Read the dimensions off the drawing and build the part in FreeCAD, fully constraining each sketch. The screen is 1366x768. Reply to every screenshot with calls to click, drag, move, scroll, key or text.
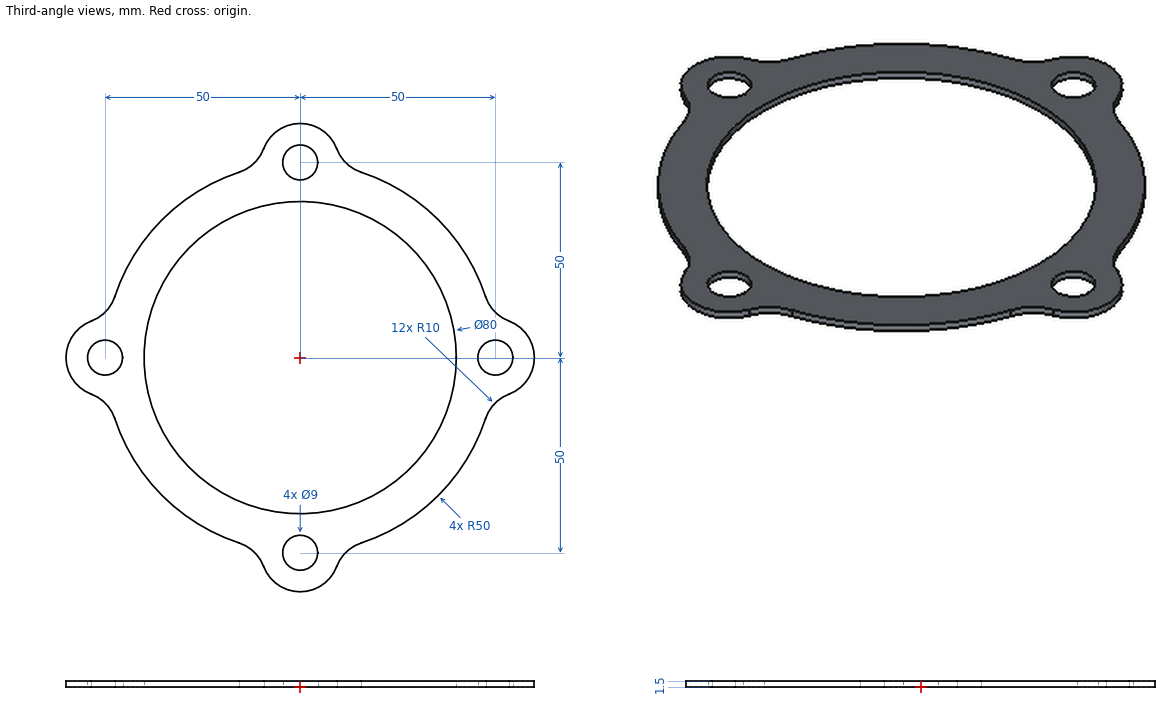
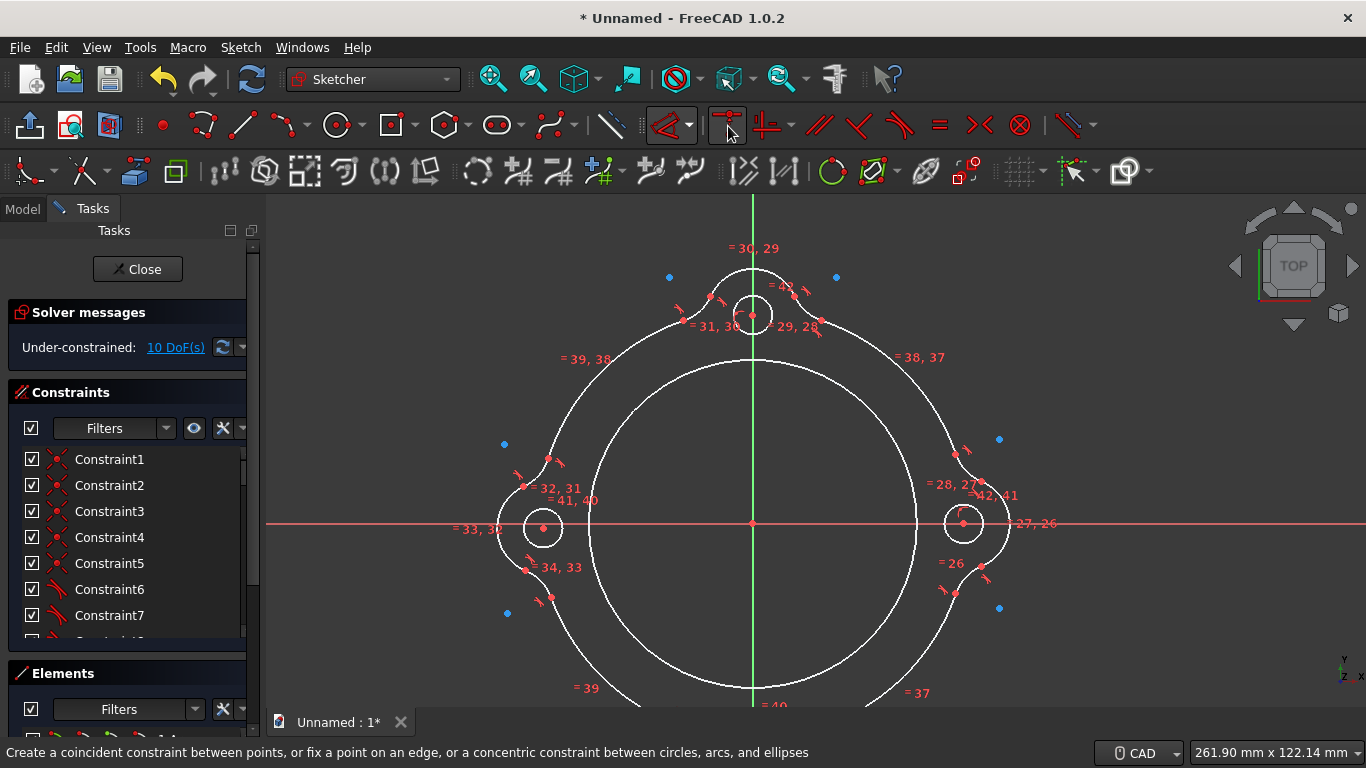
click(543, 528)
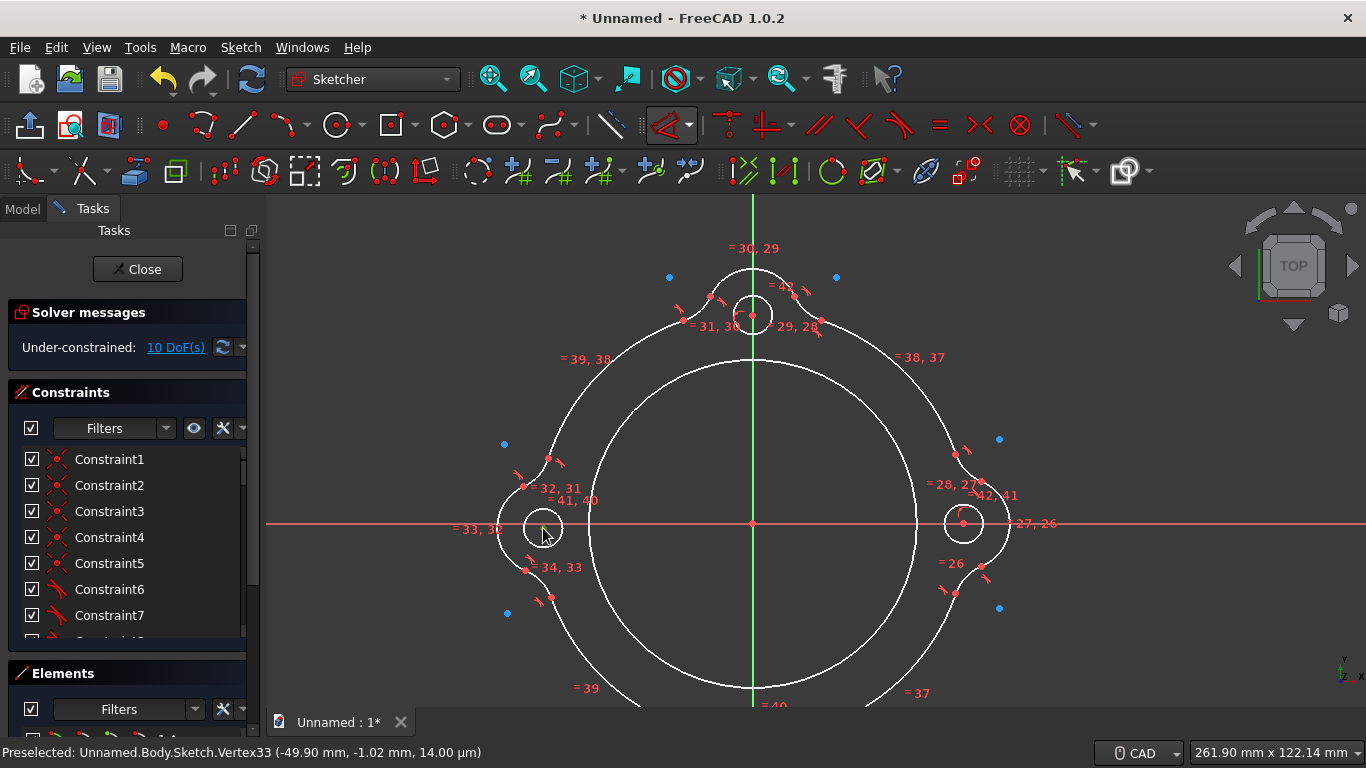
click(359, 524)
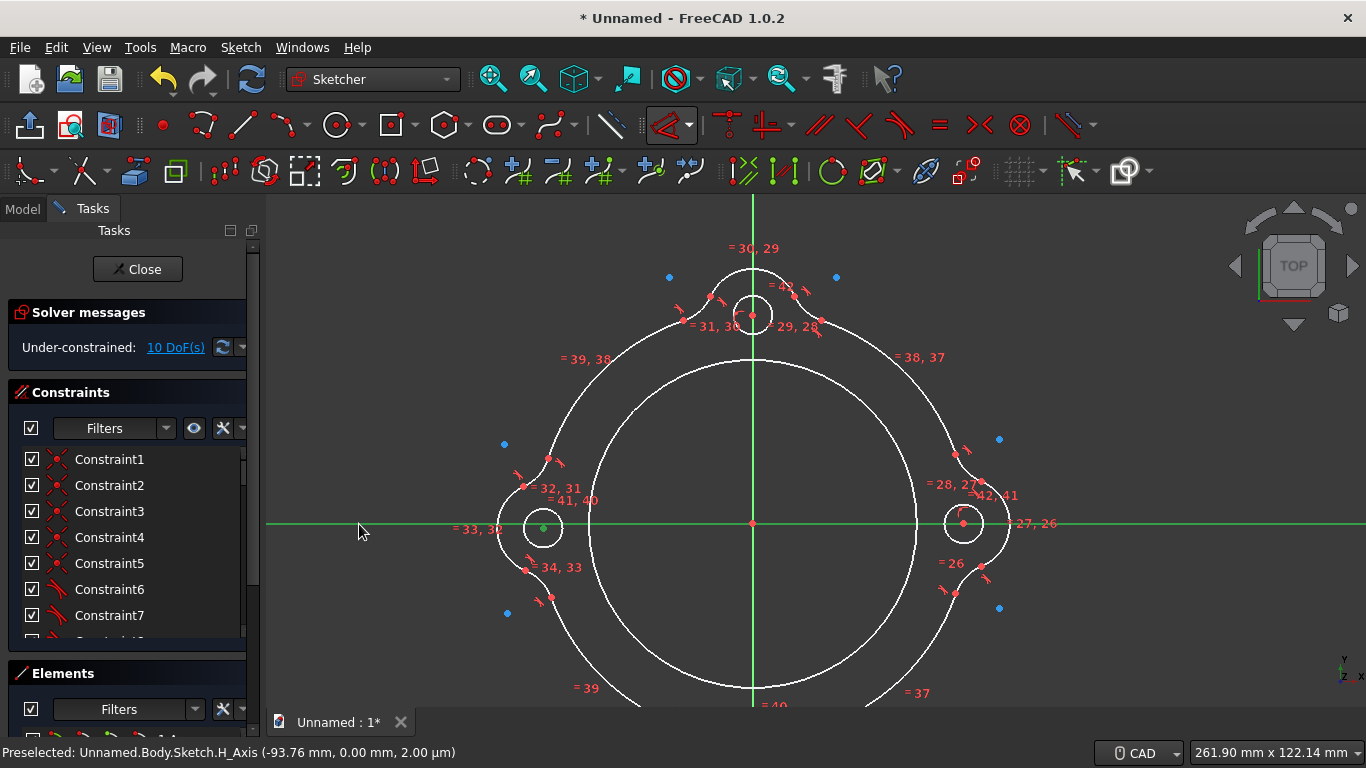
click(728, 126)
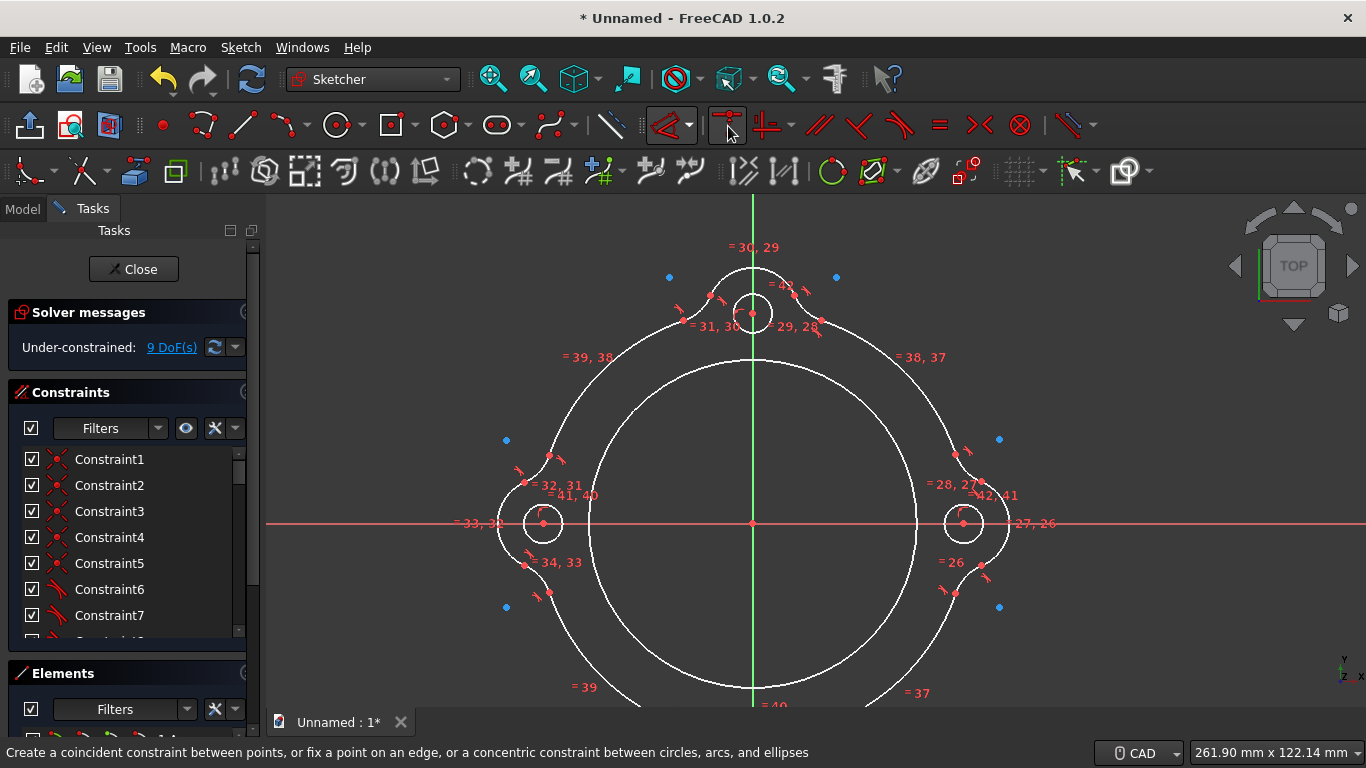
scroll(737, 301, down, 2)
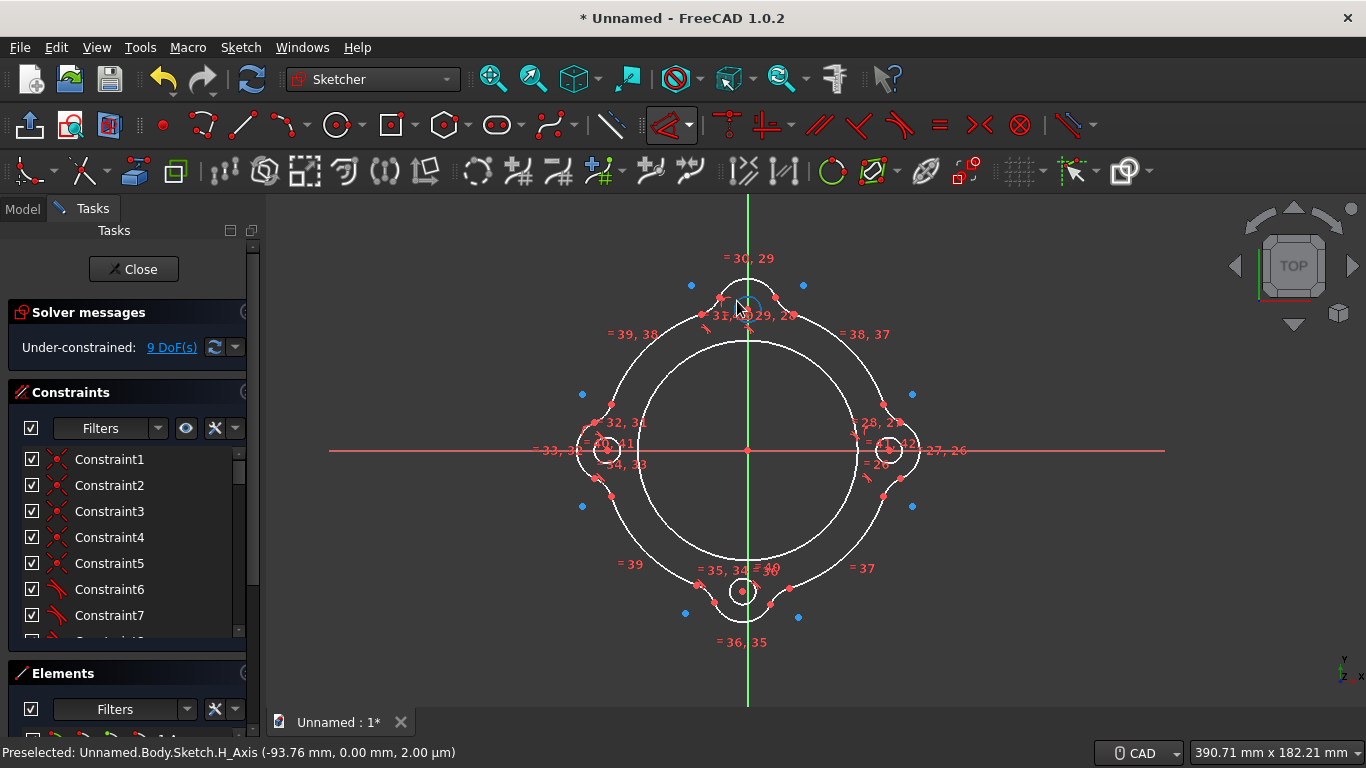
click(743, 592)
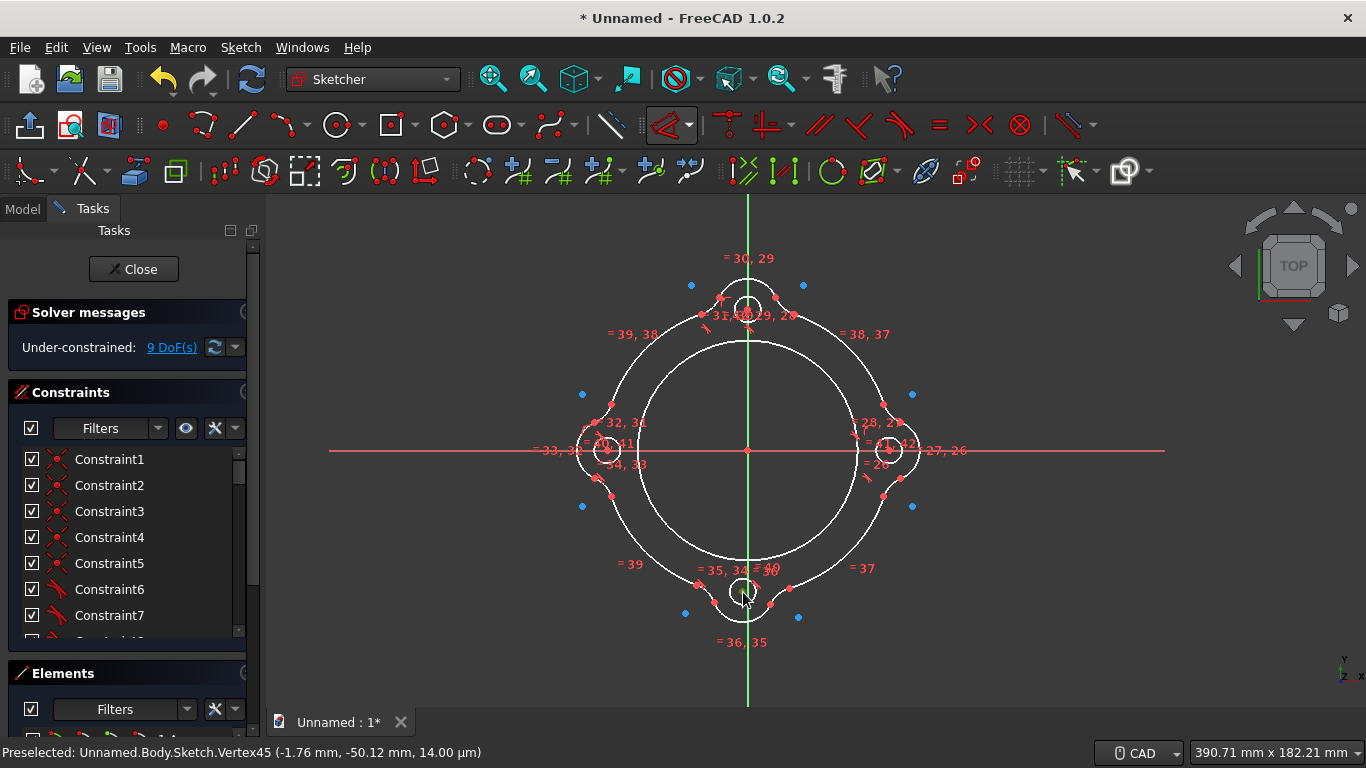
click(748, 516)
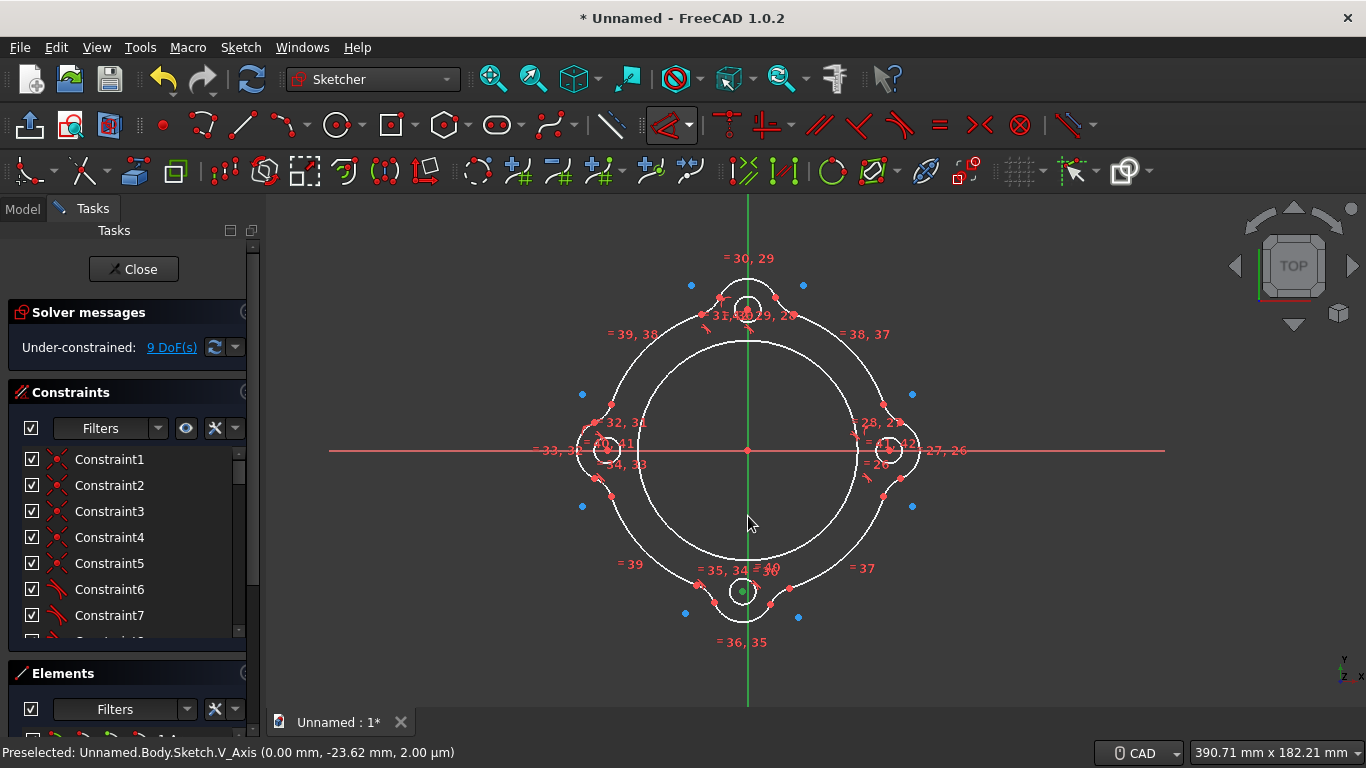
click(728, 126)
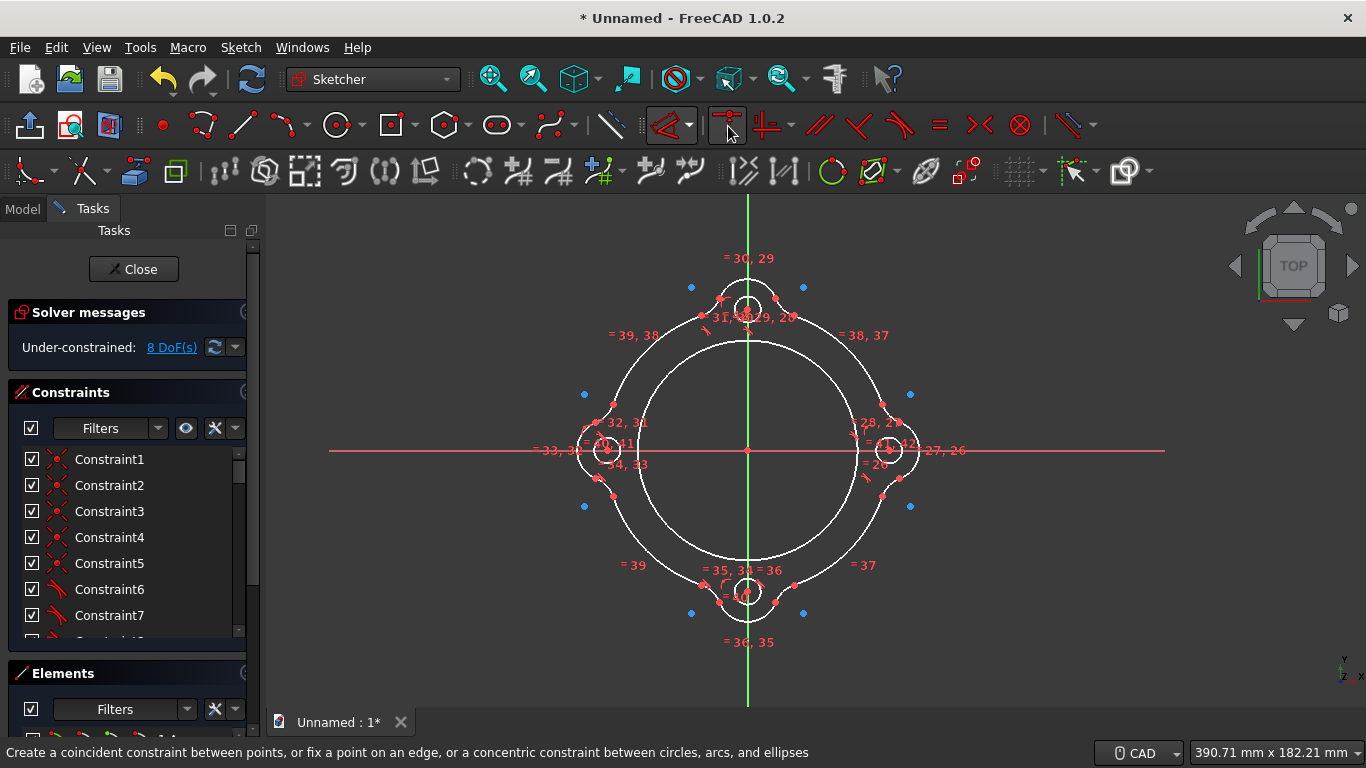
click(666, 126)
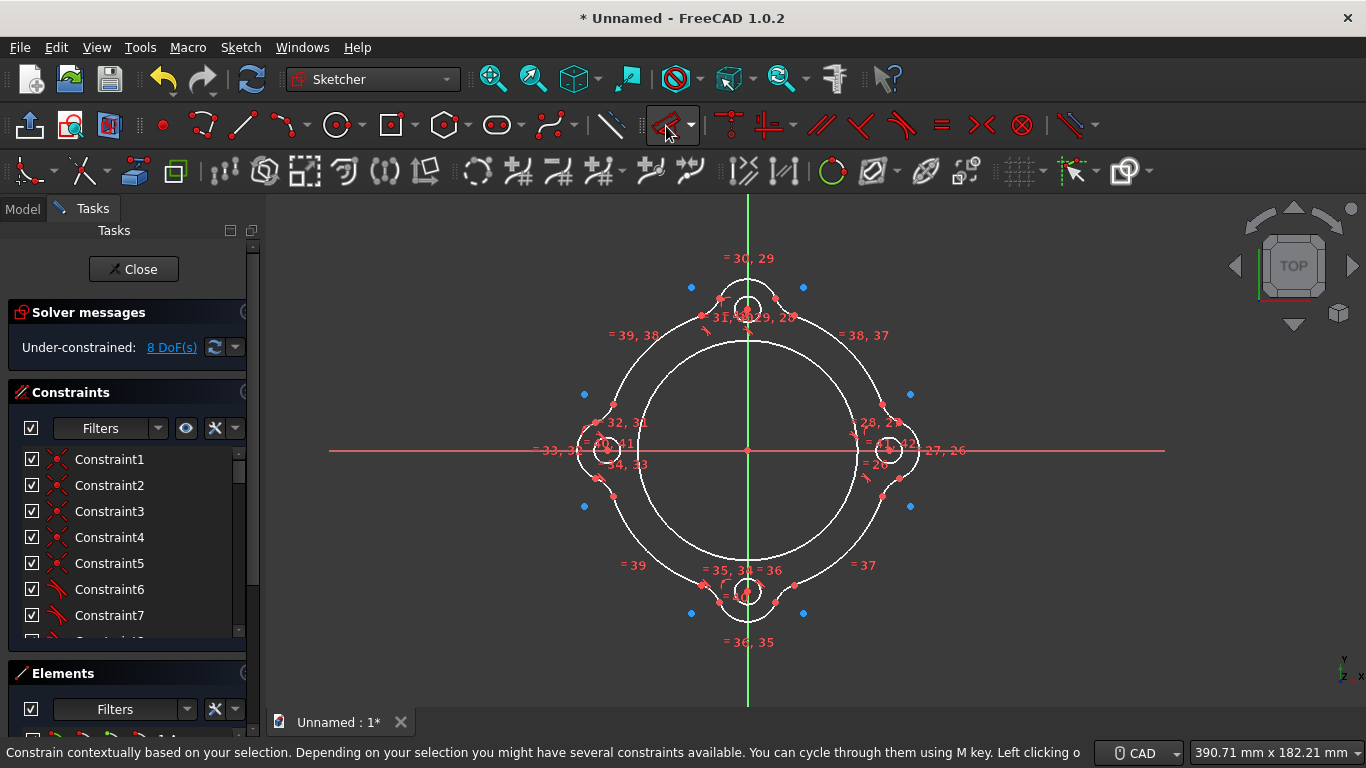
click(829, 568)
click(847, 594)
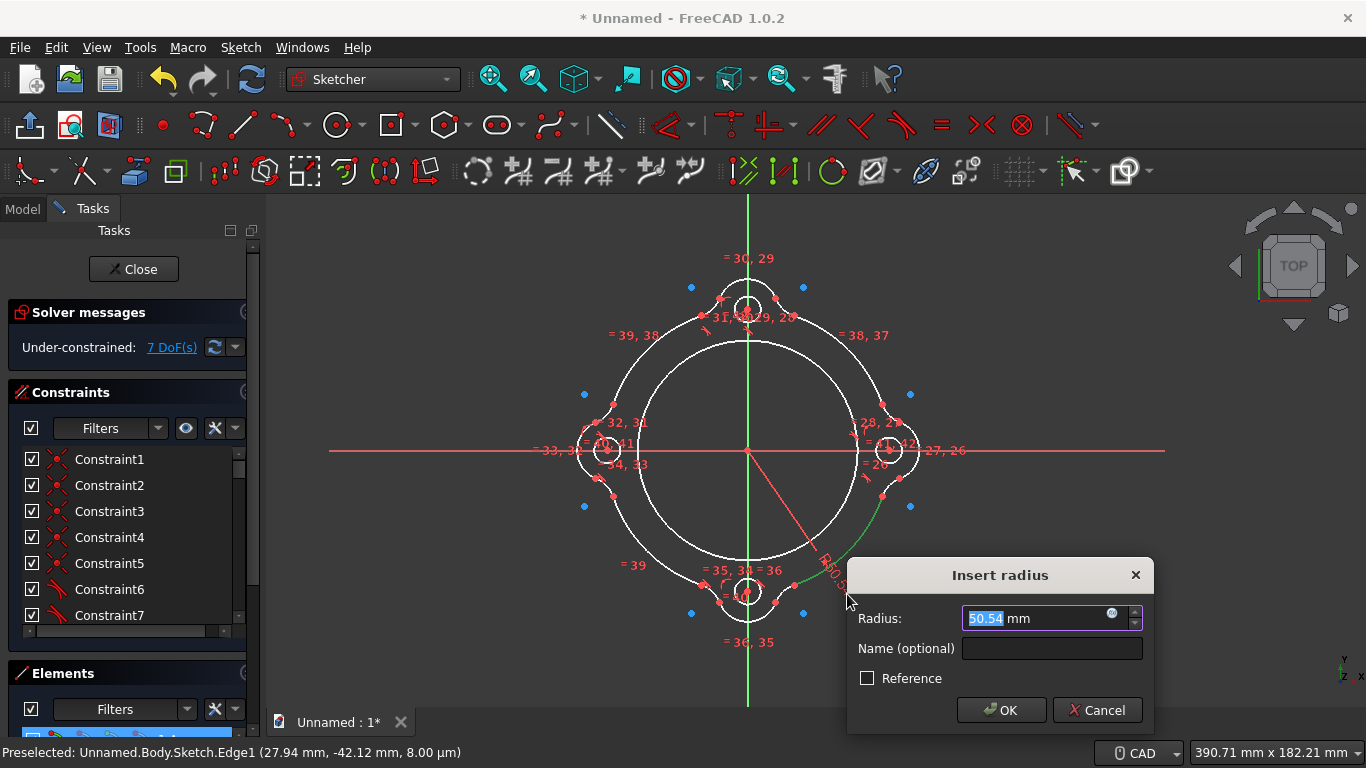
text(50)
key(Return)